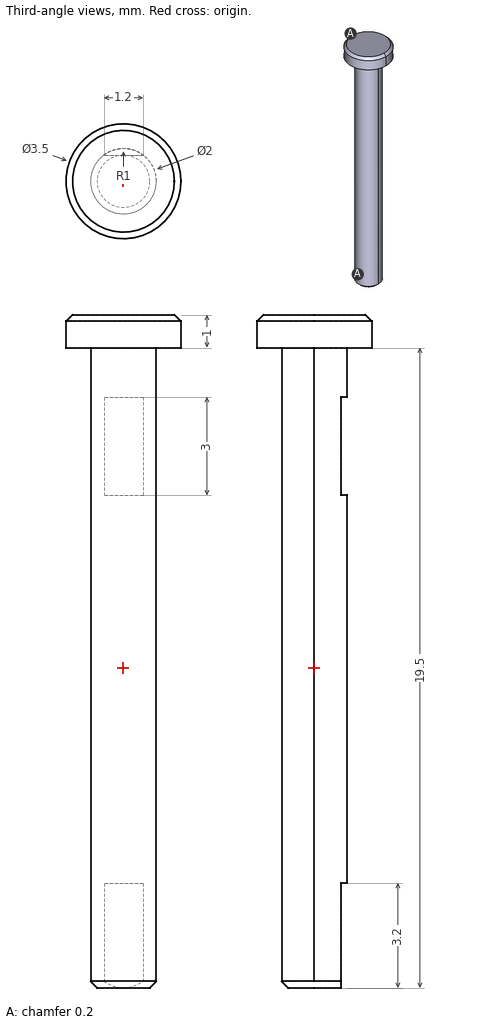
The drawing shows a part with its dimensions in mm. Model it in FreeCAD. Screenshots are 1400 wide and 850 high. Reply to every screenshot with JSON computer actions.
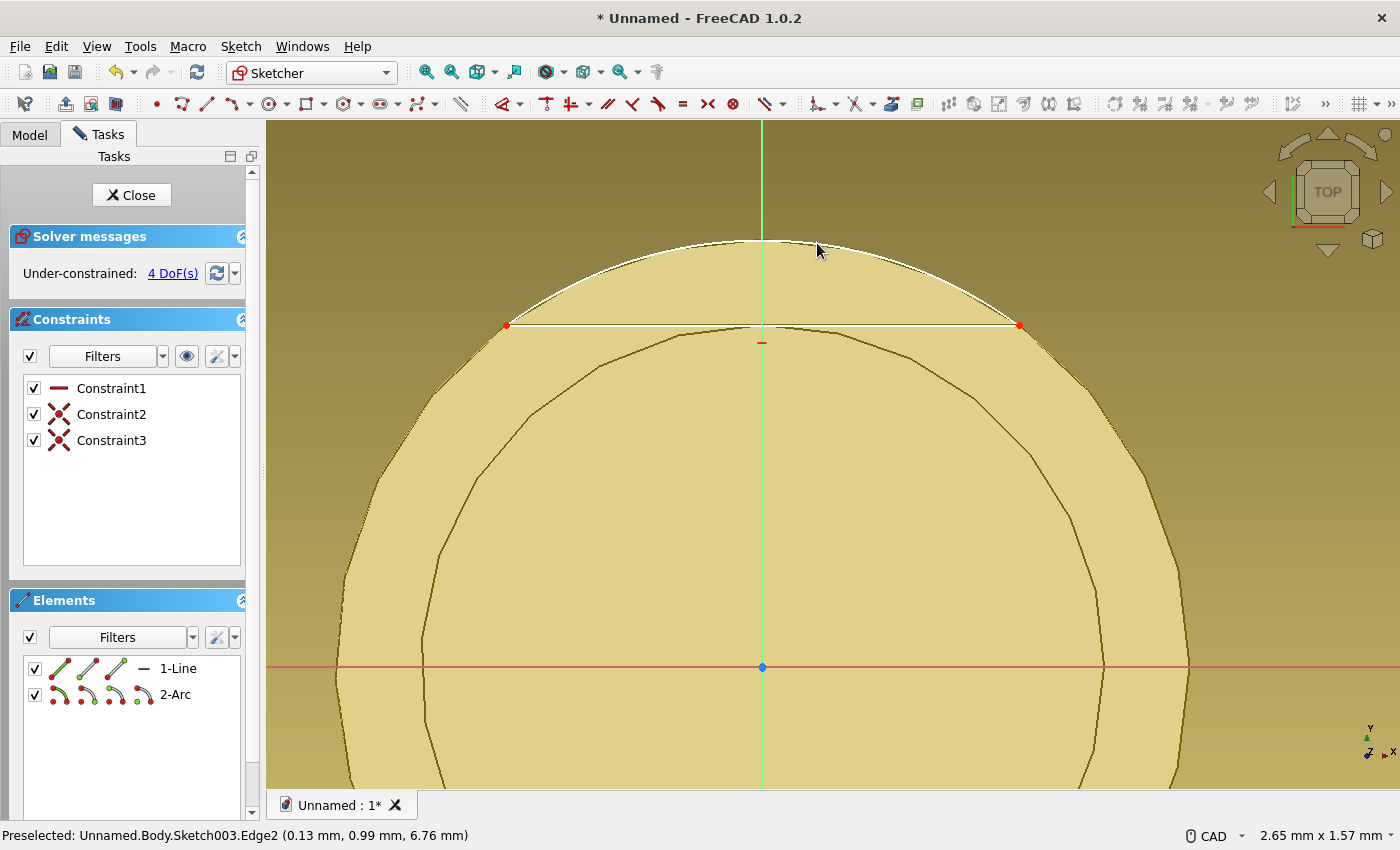
{"action": "left_click_drag", "start_coordinate": [752, 657], "coordinate": [773, 678]}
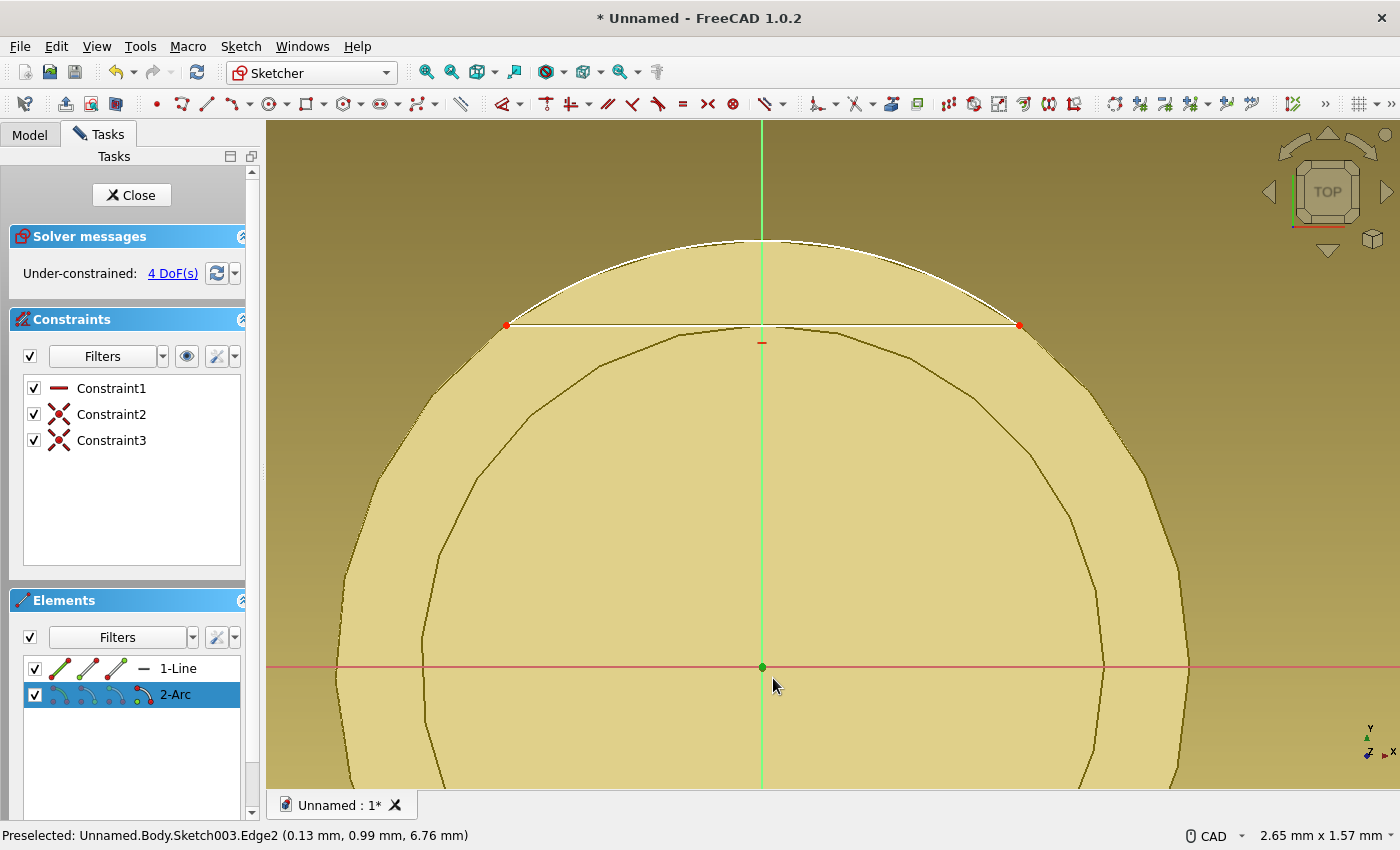
{"action": "key", "text": "c"}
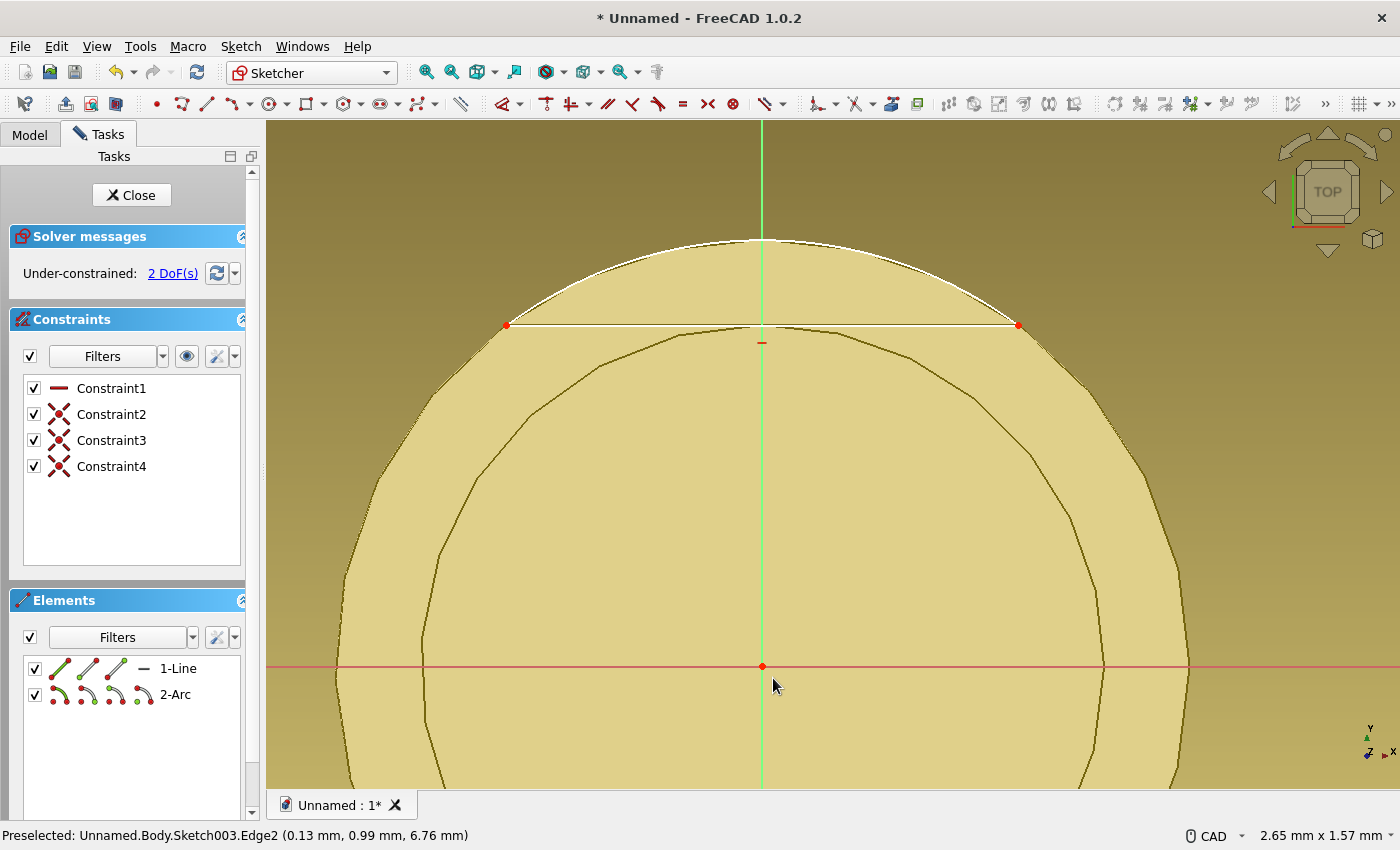
{"action": "left_click", "coordinate": [871, 254]}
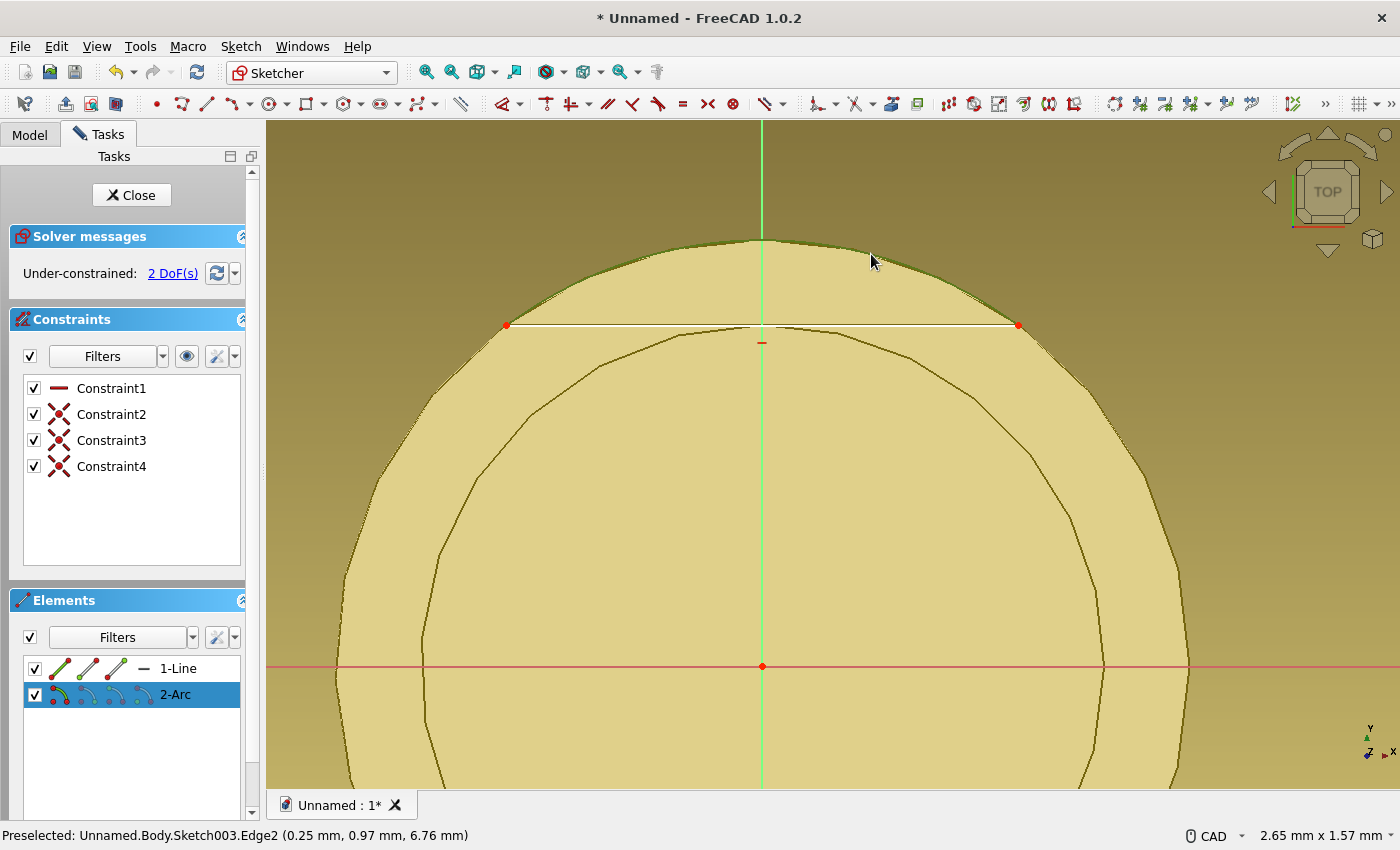
{"action": "key", "text": "k r"}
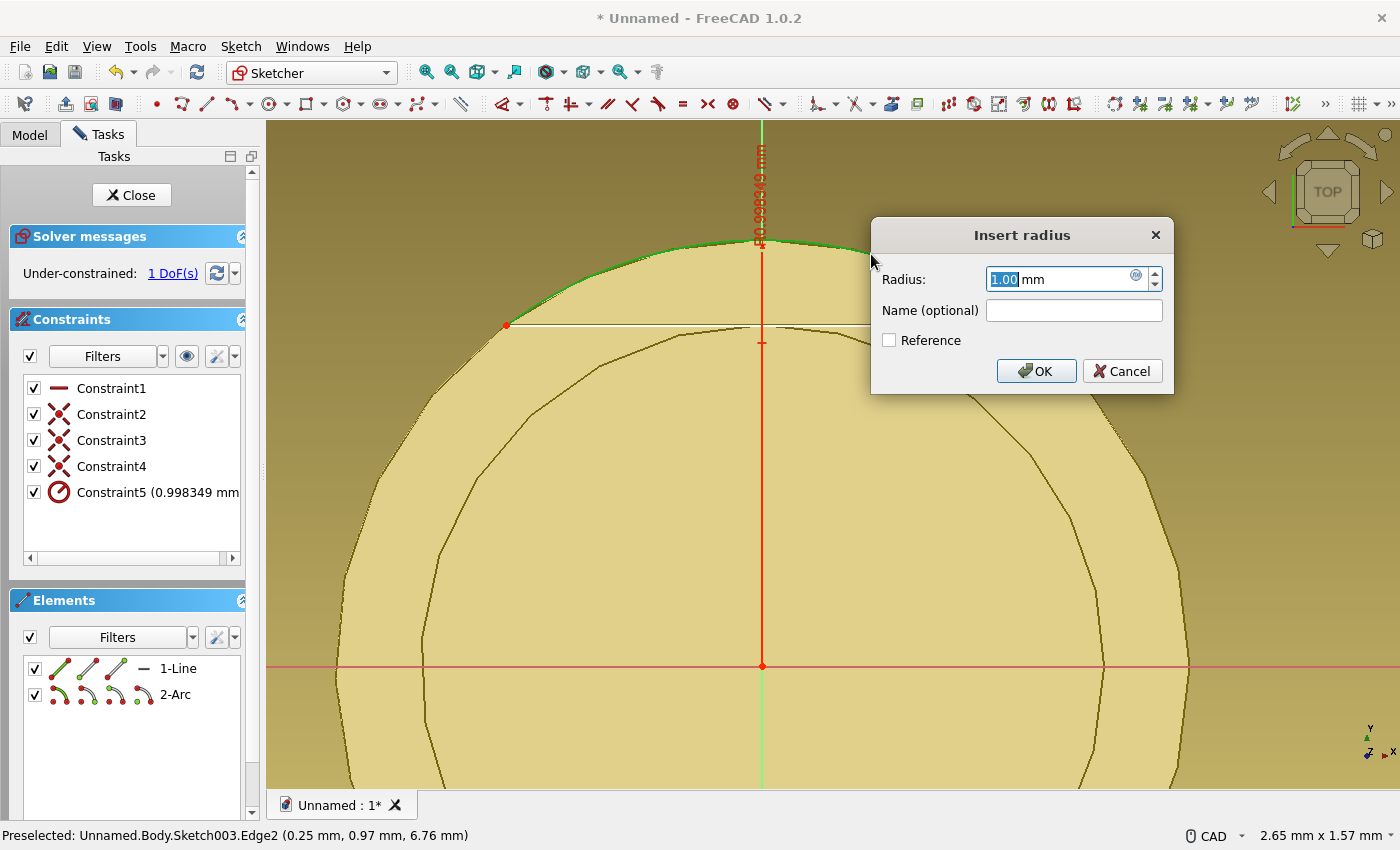
{"action": "type", "text": "1"}
{"action": "key", "text": "Return"}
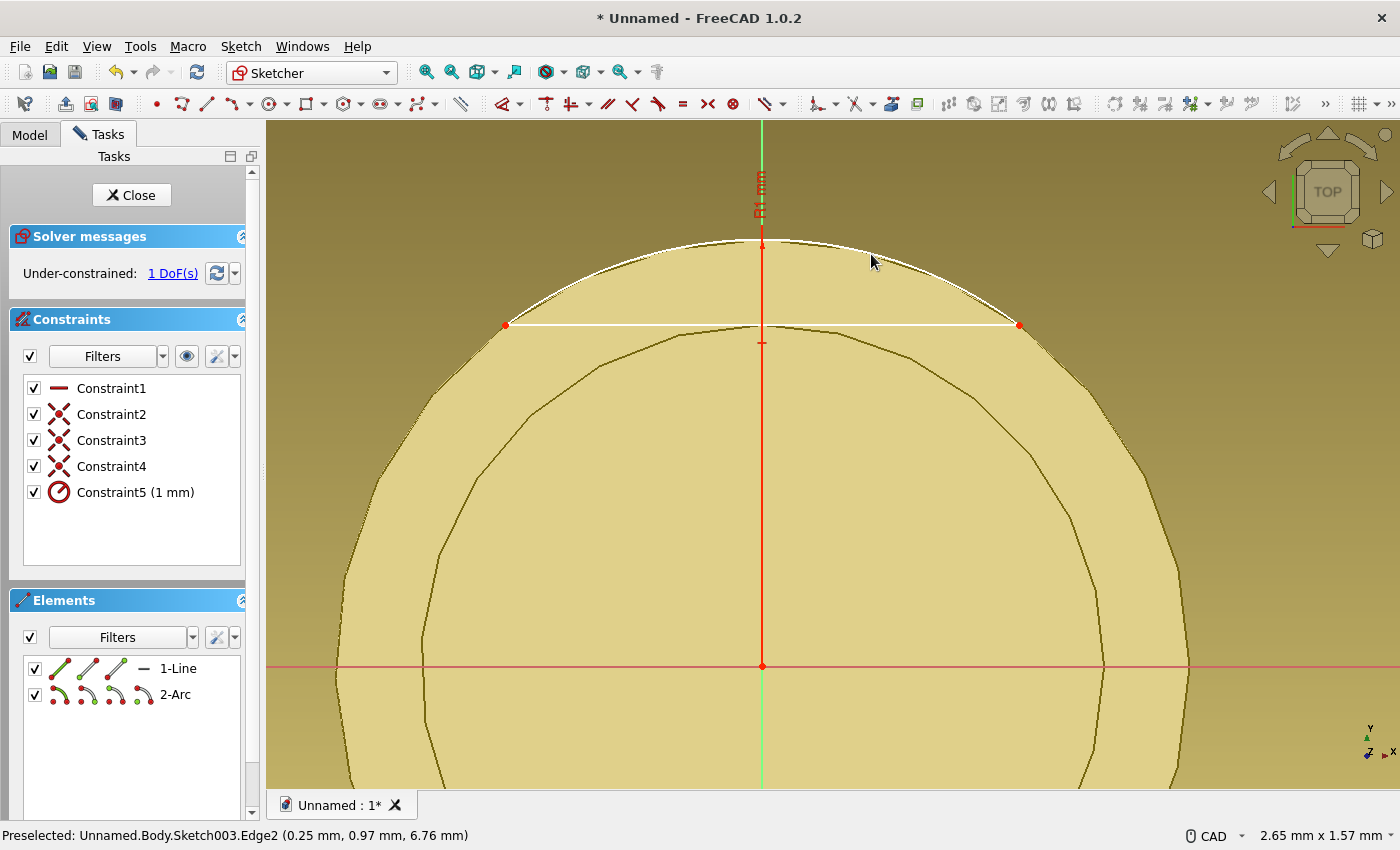
{"action": "left_click", "coordinate": [865, 325]}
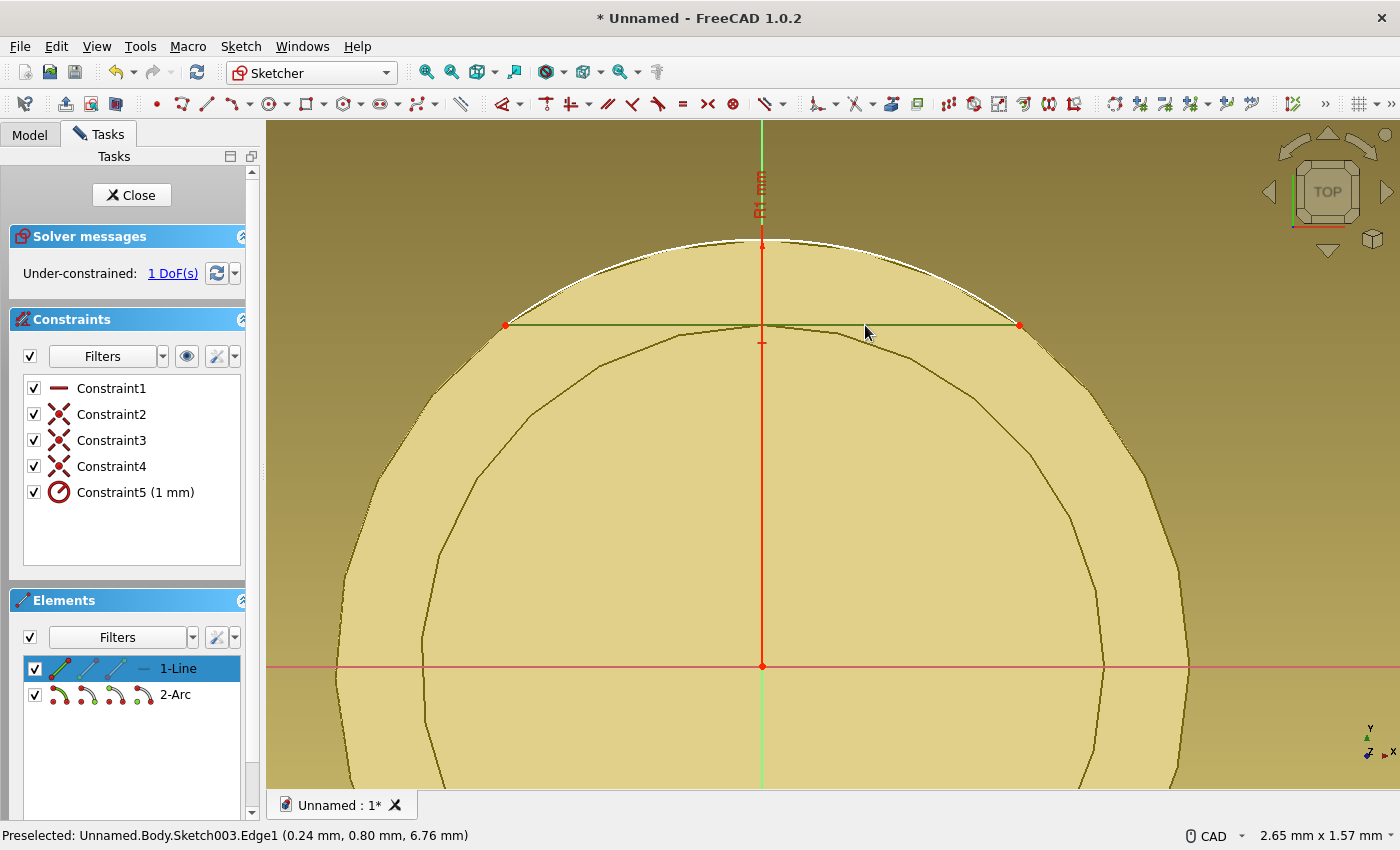
{"action": "key", "text": "l"}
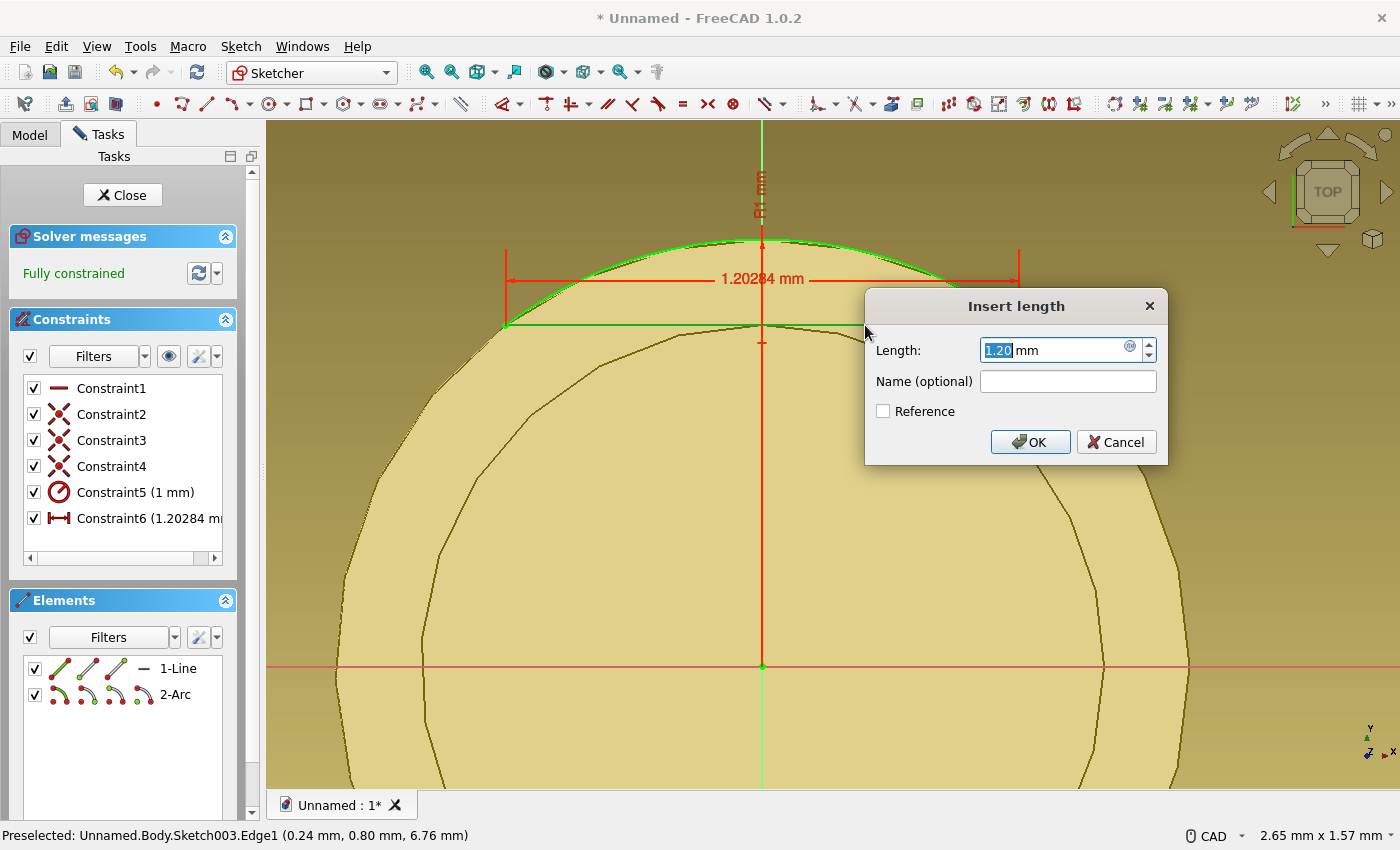
{"action": "type", "text": "1.2"}
{"action": "key", "text": "Return"}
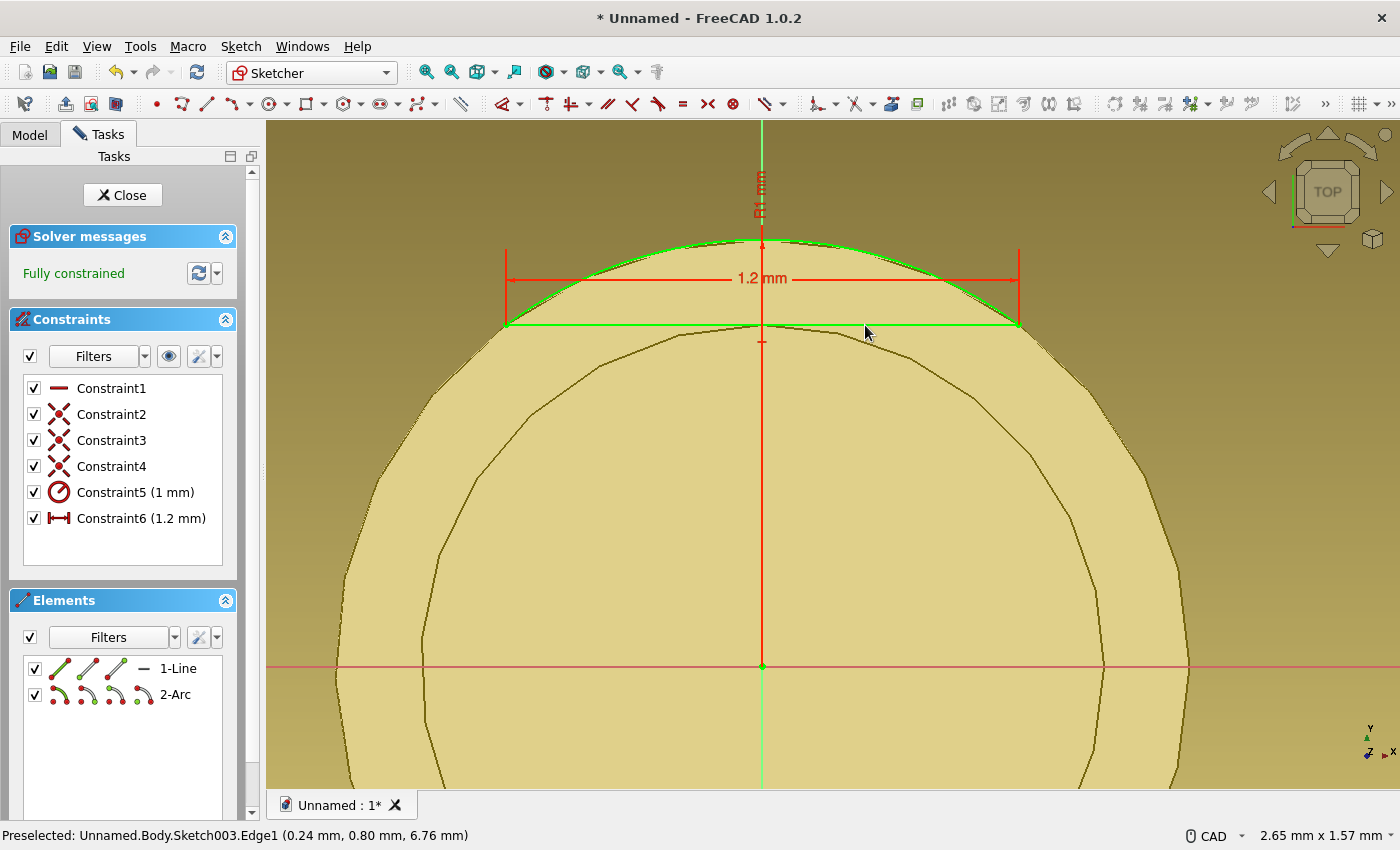
{"action": "left_click", "coordinate": [123, 195]}